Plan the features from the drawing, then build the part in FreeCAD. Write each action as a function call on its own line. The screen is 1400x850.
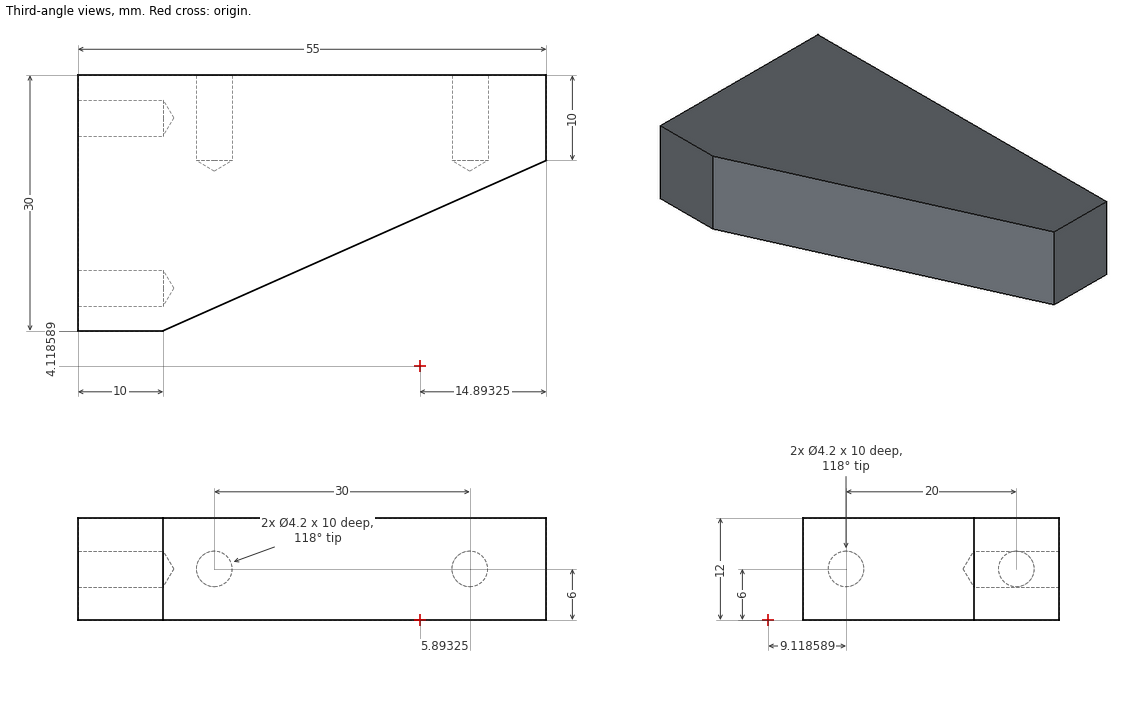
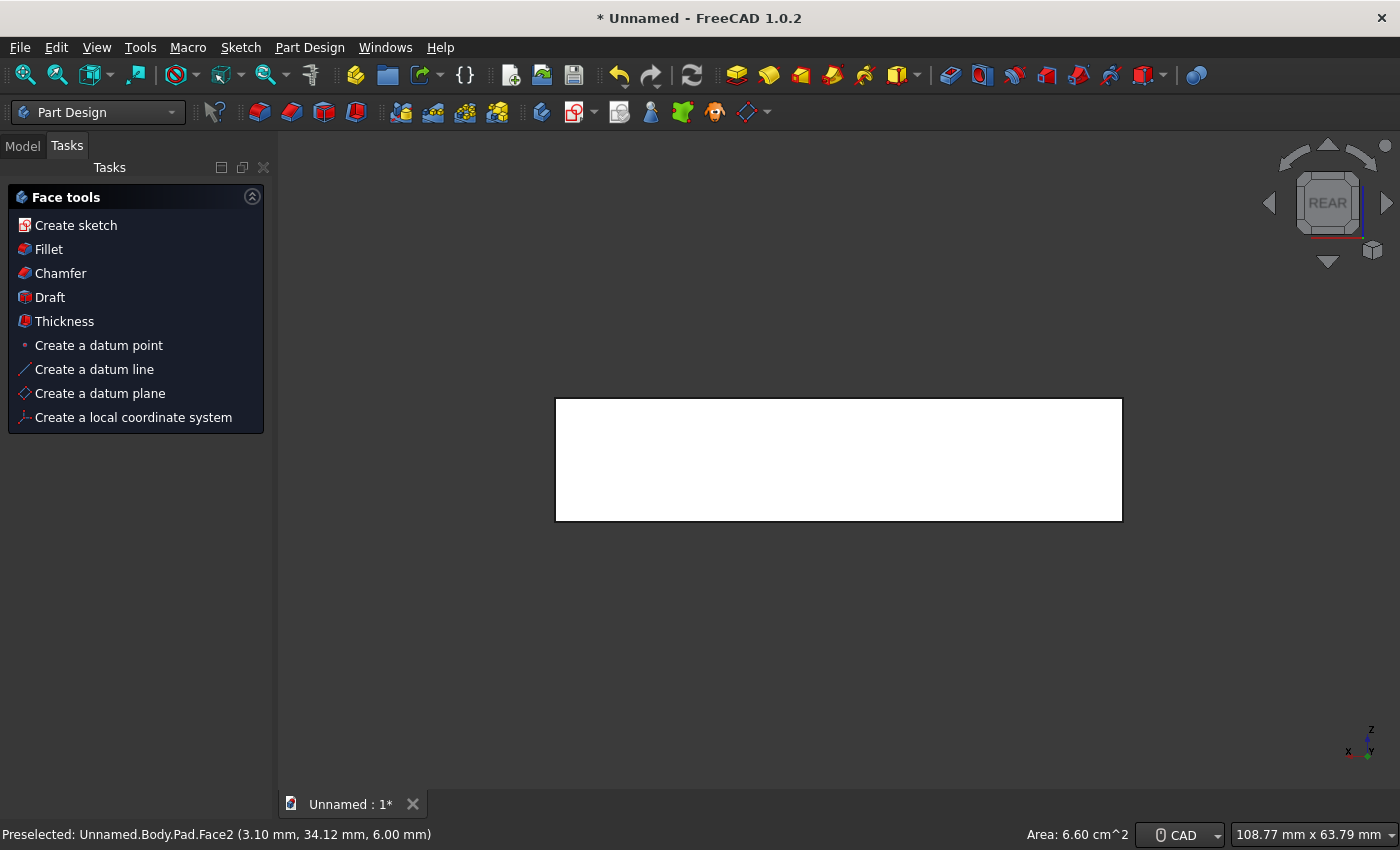
click(574, 112)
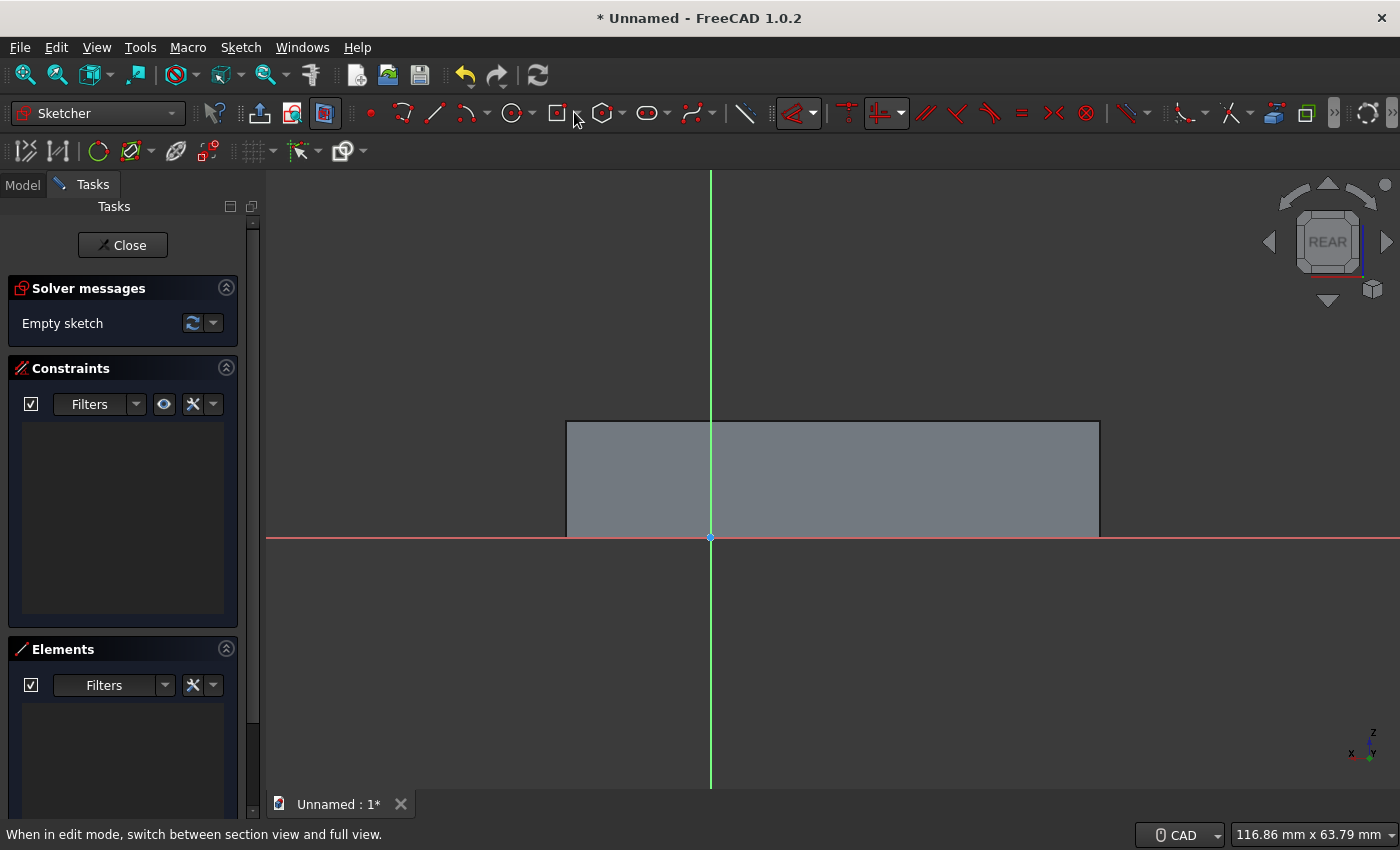
scroll(841, 521, up, 3)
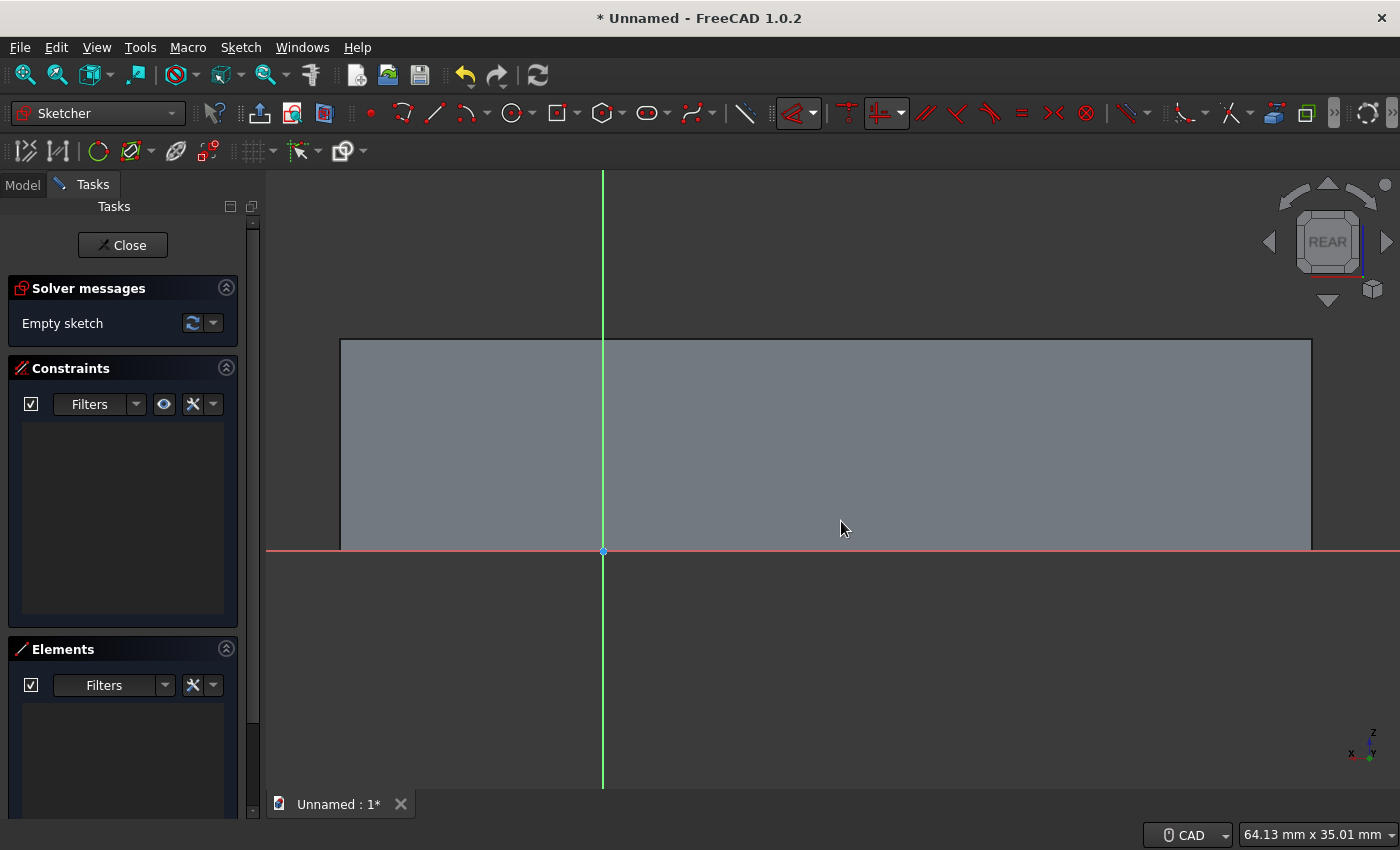
click(512, 114)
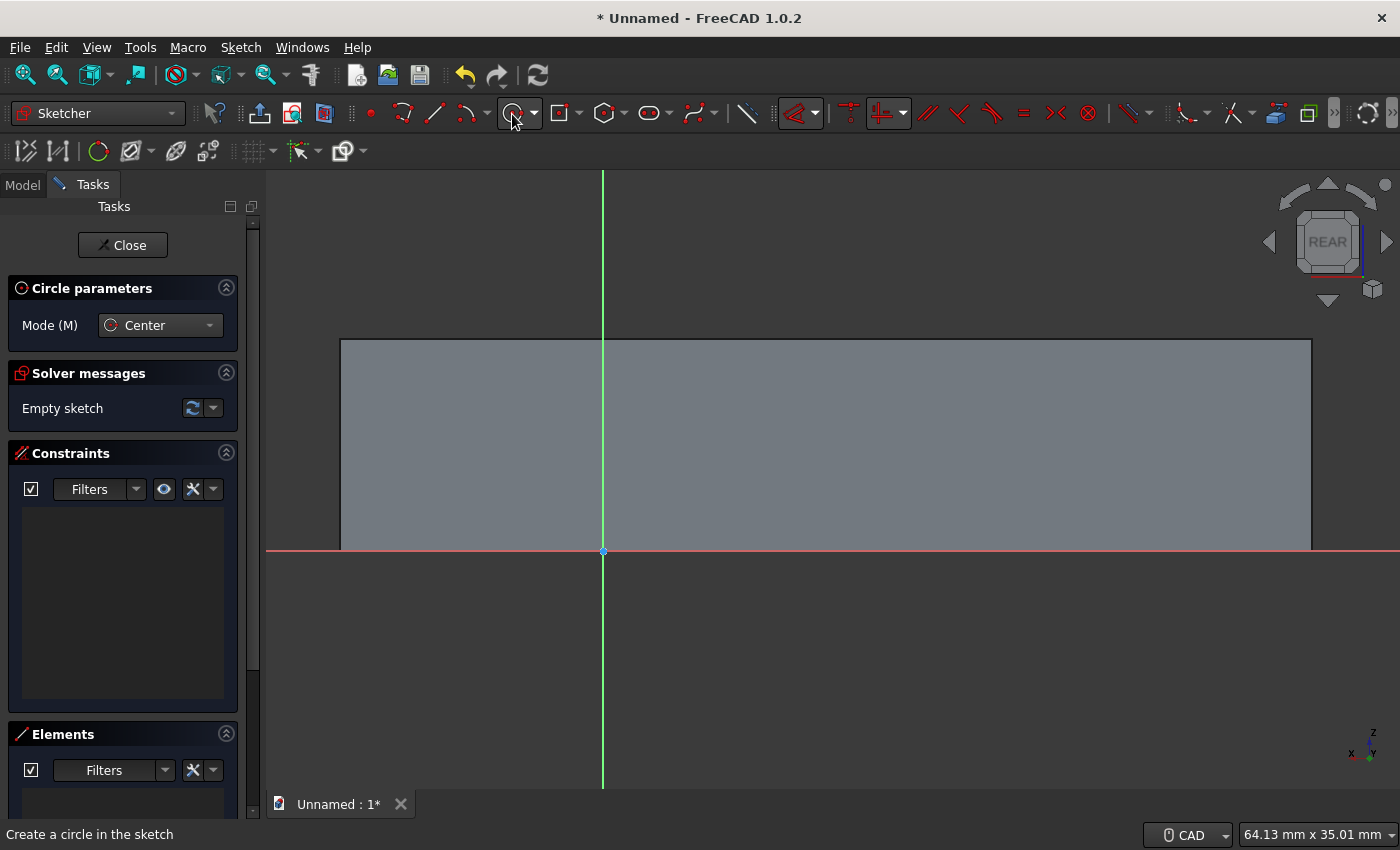
click(1029, 445)
click(1056, 419)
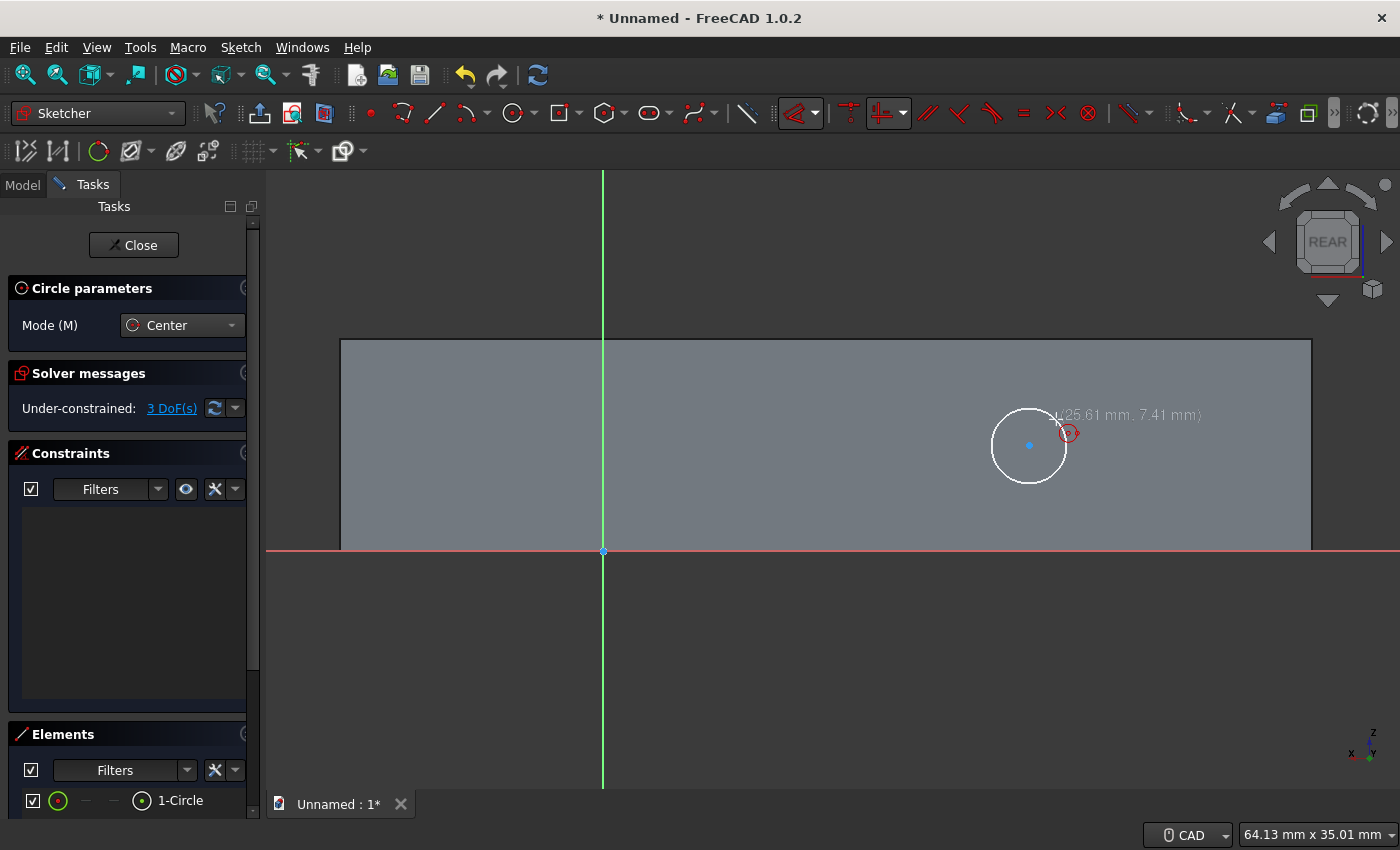
click(499, 445)
click(525, 419)
key(Escape)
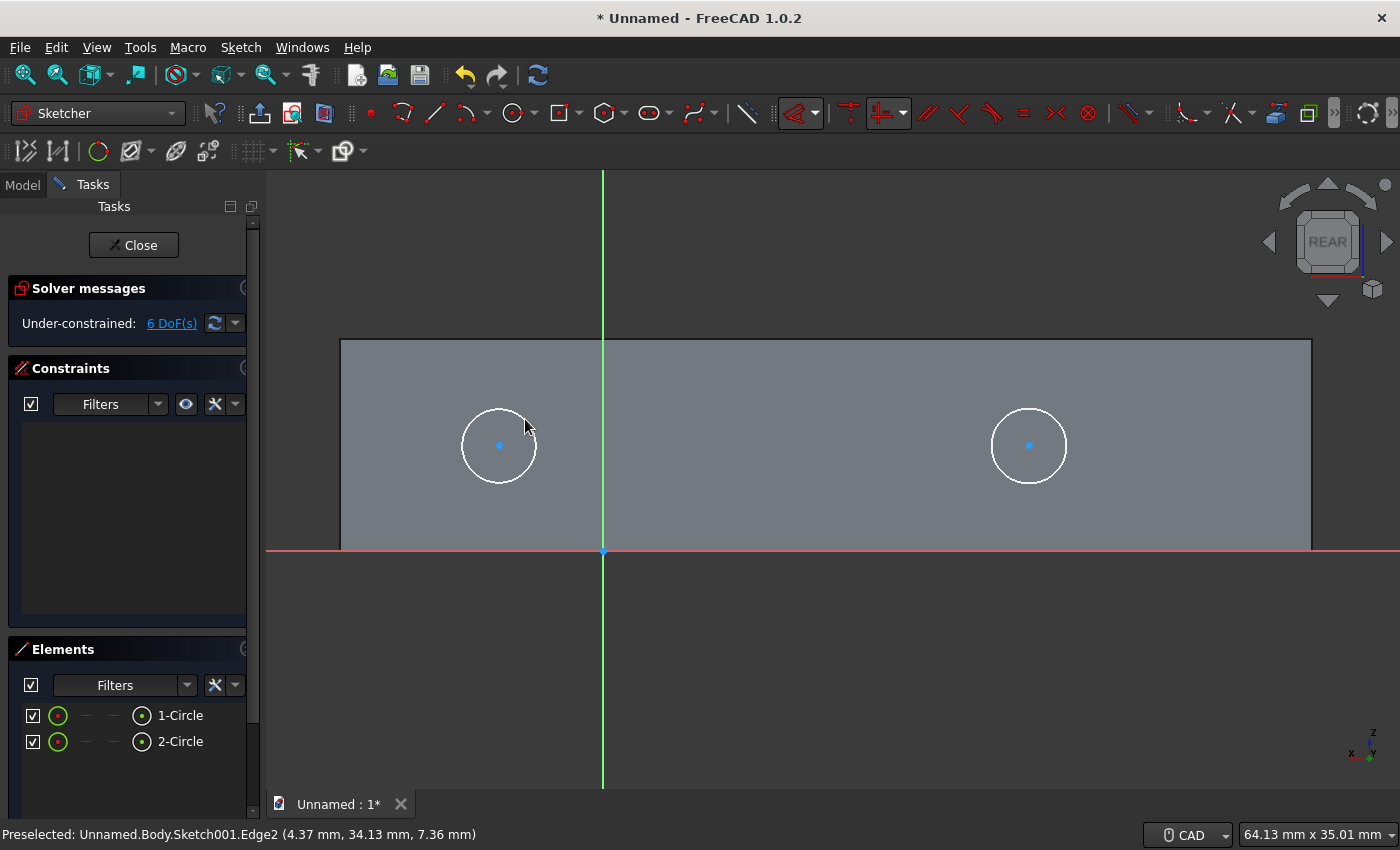
click(1055, 419)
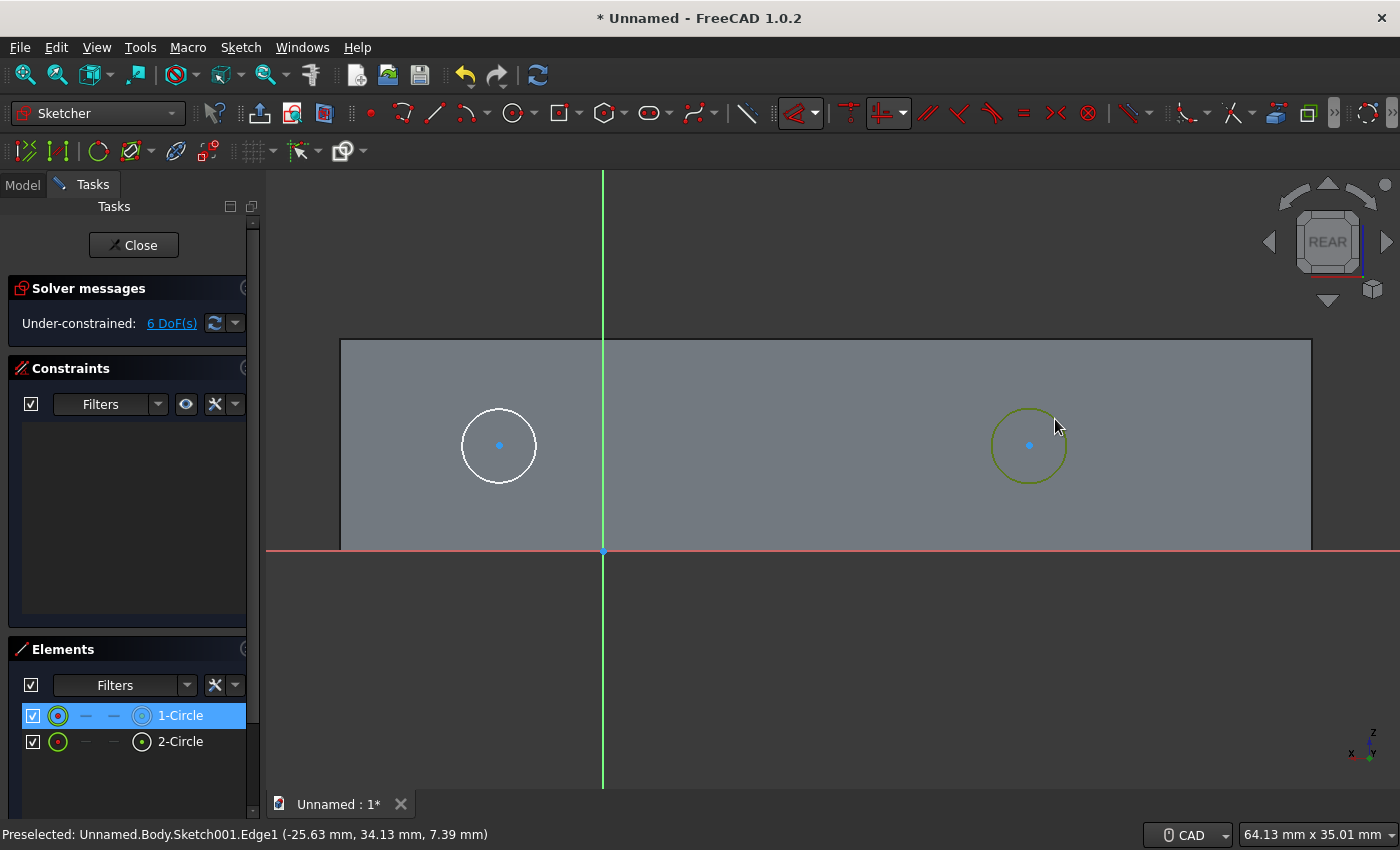
click(525, 420)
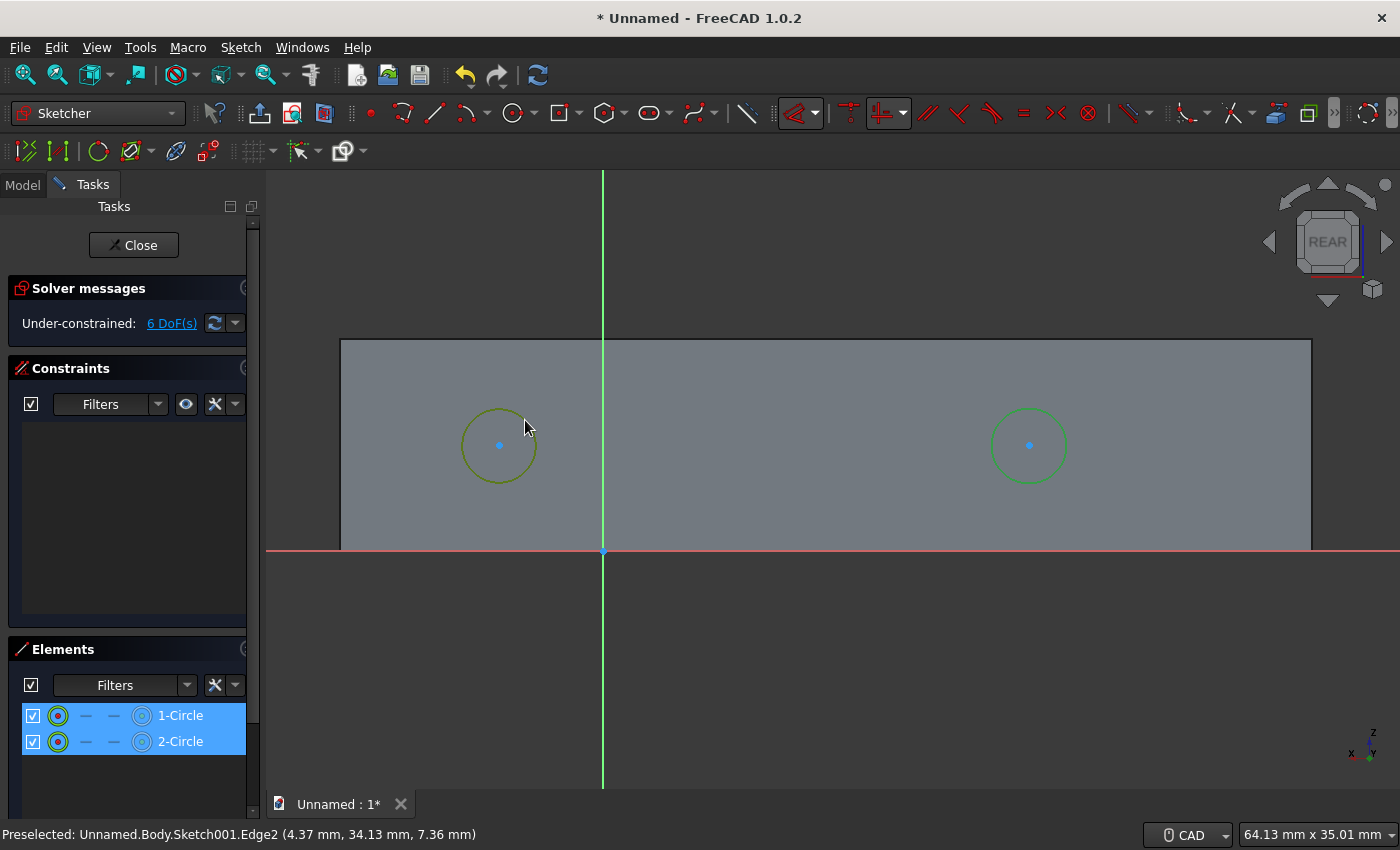
click(1024, 114)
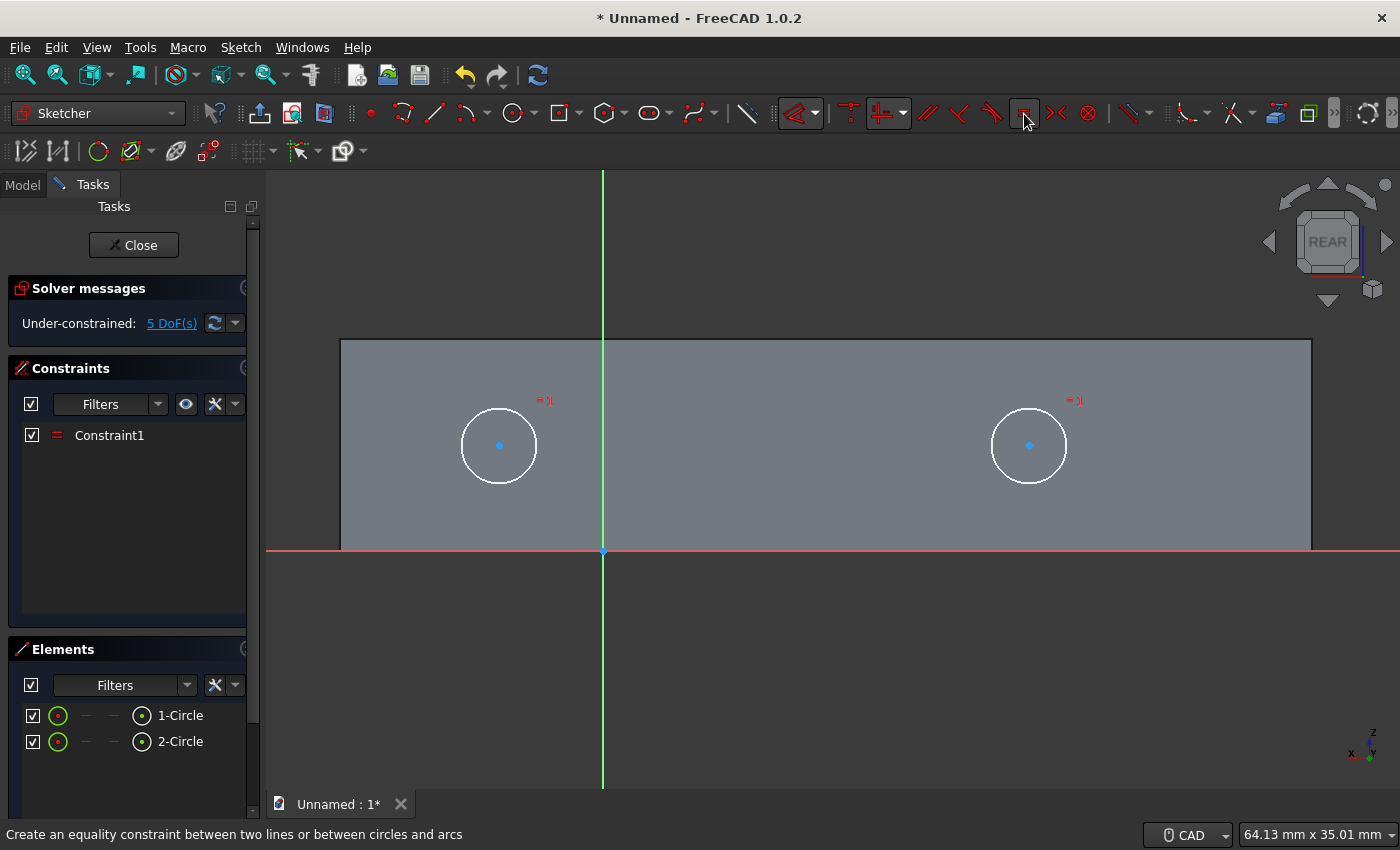
click(1055, 419)